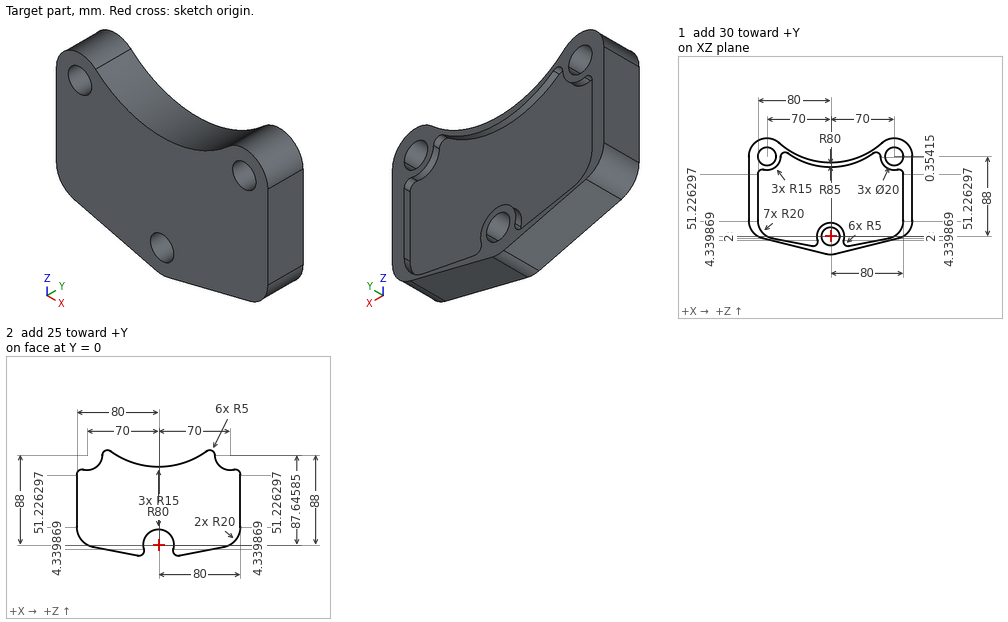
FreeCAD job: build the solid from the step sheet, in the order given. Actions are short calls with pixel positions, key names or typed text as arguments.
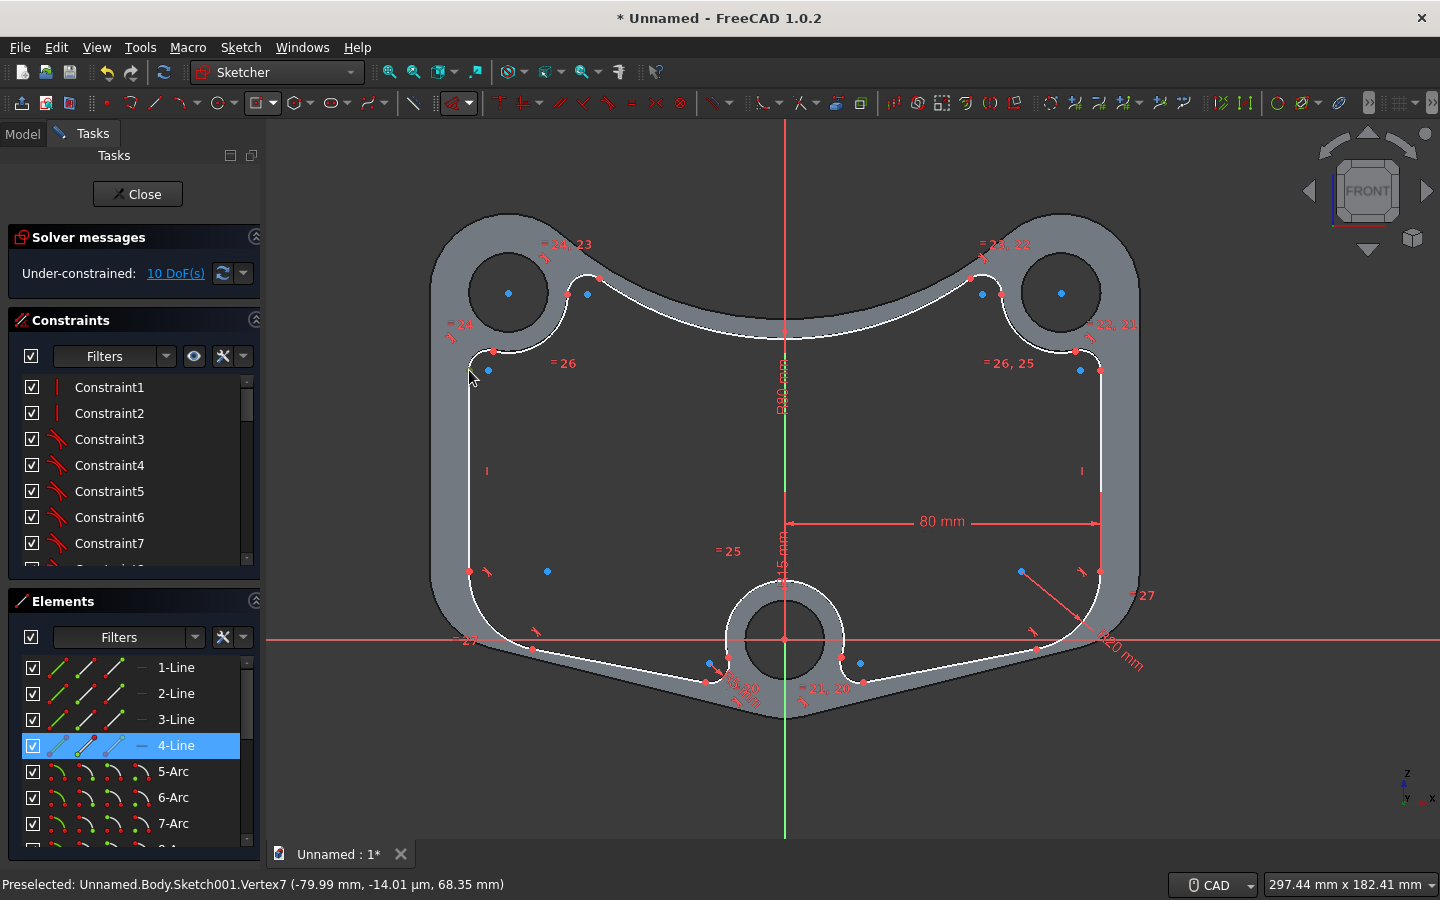
click(472, 104)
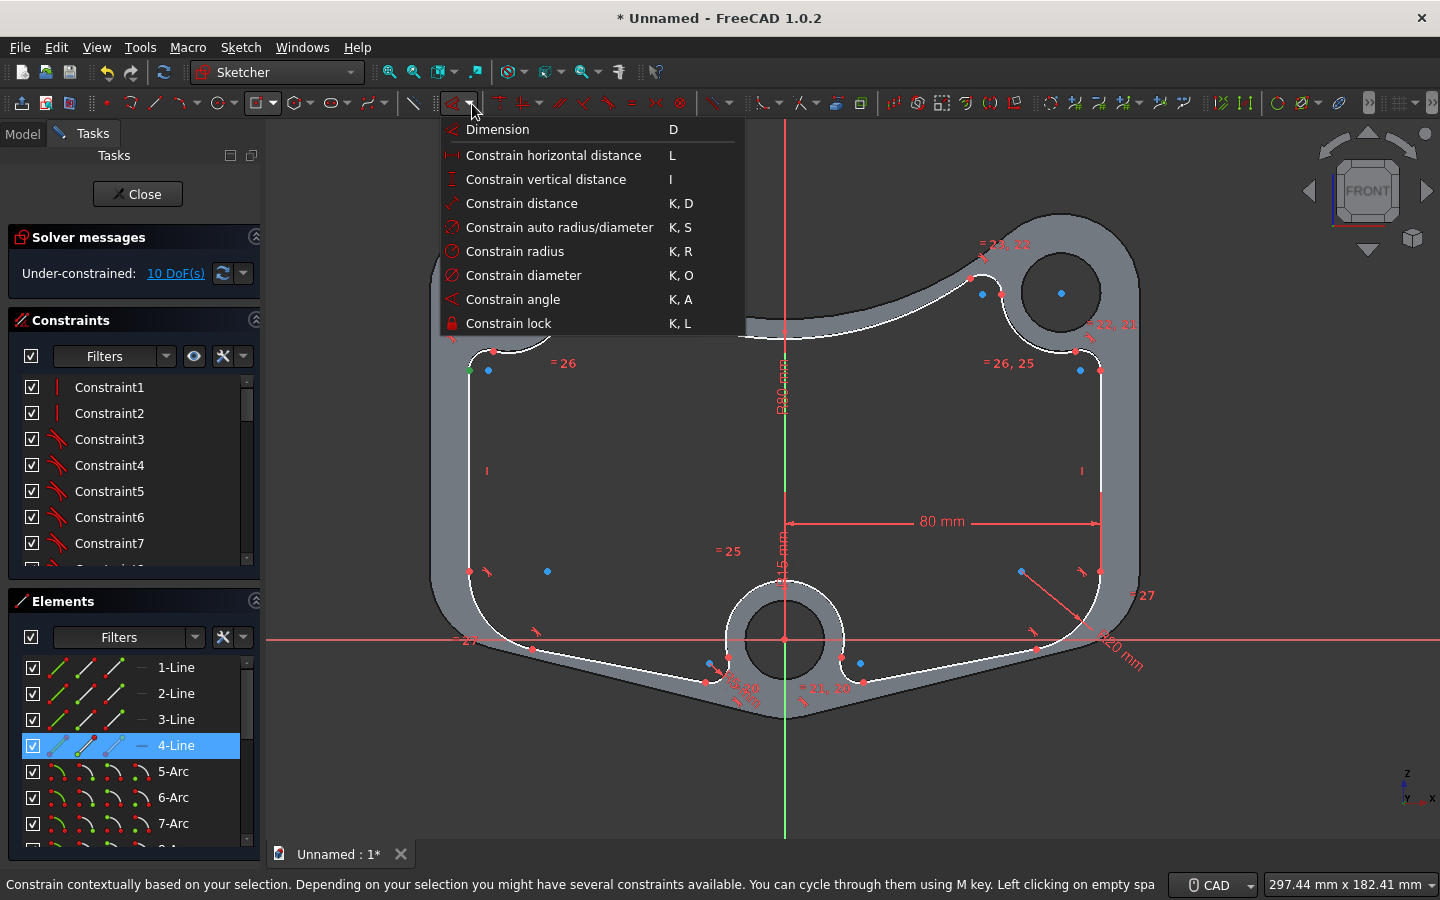
click(593, 155)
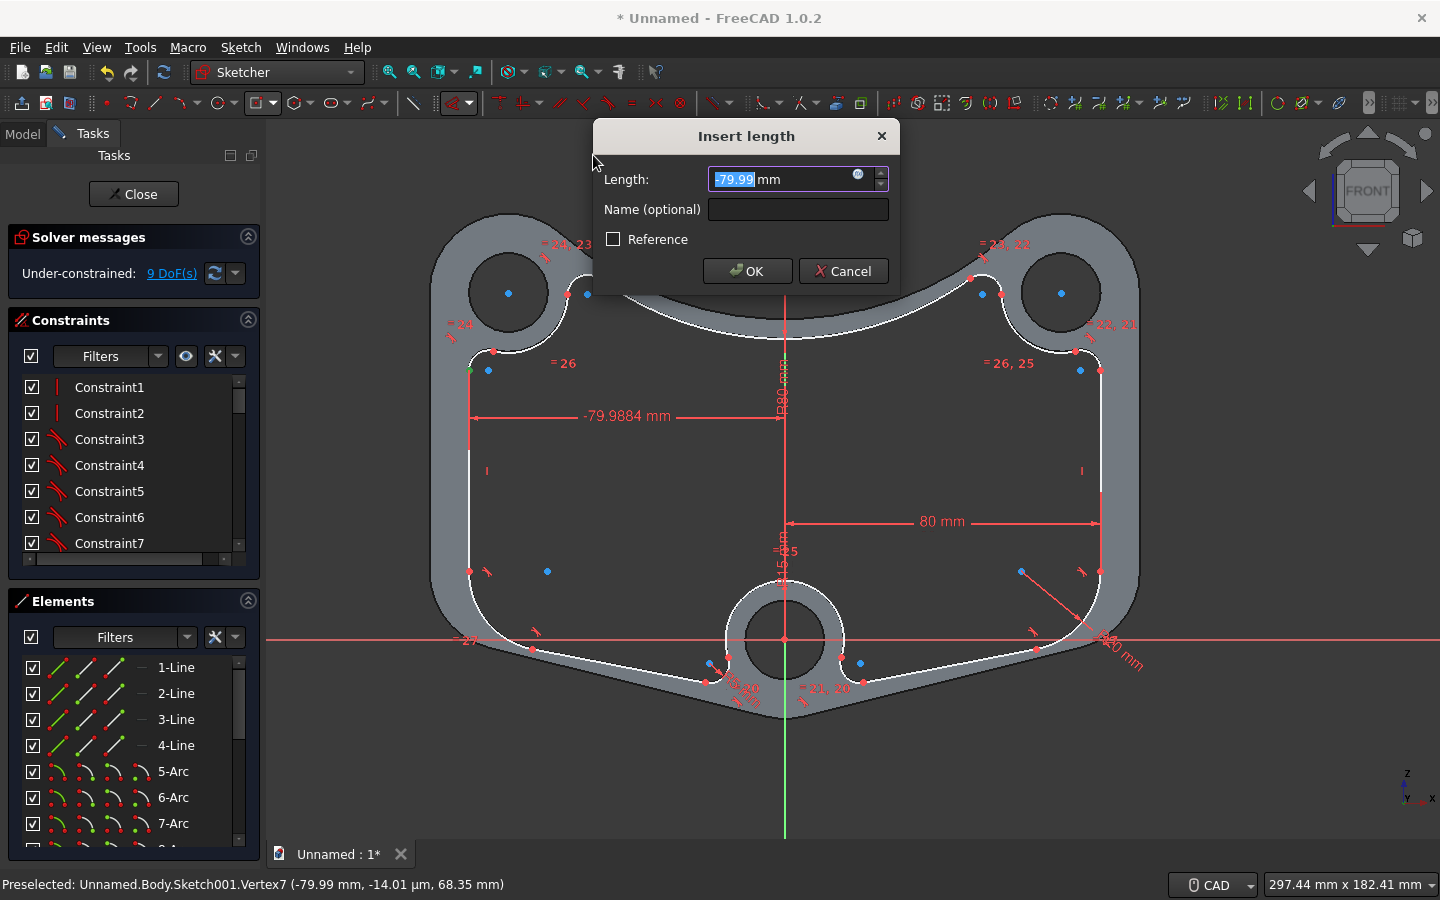
text(-80)
key(Return)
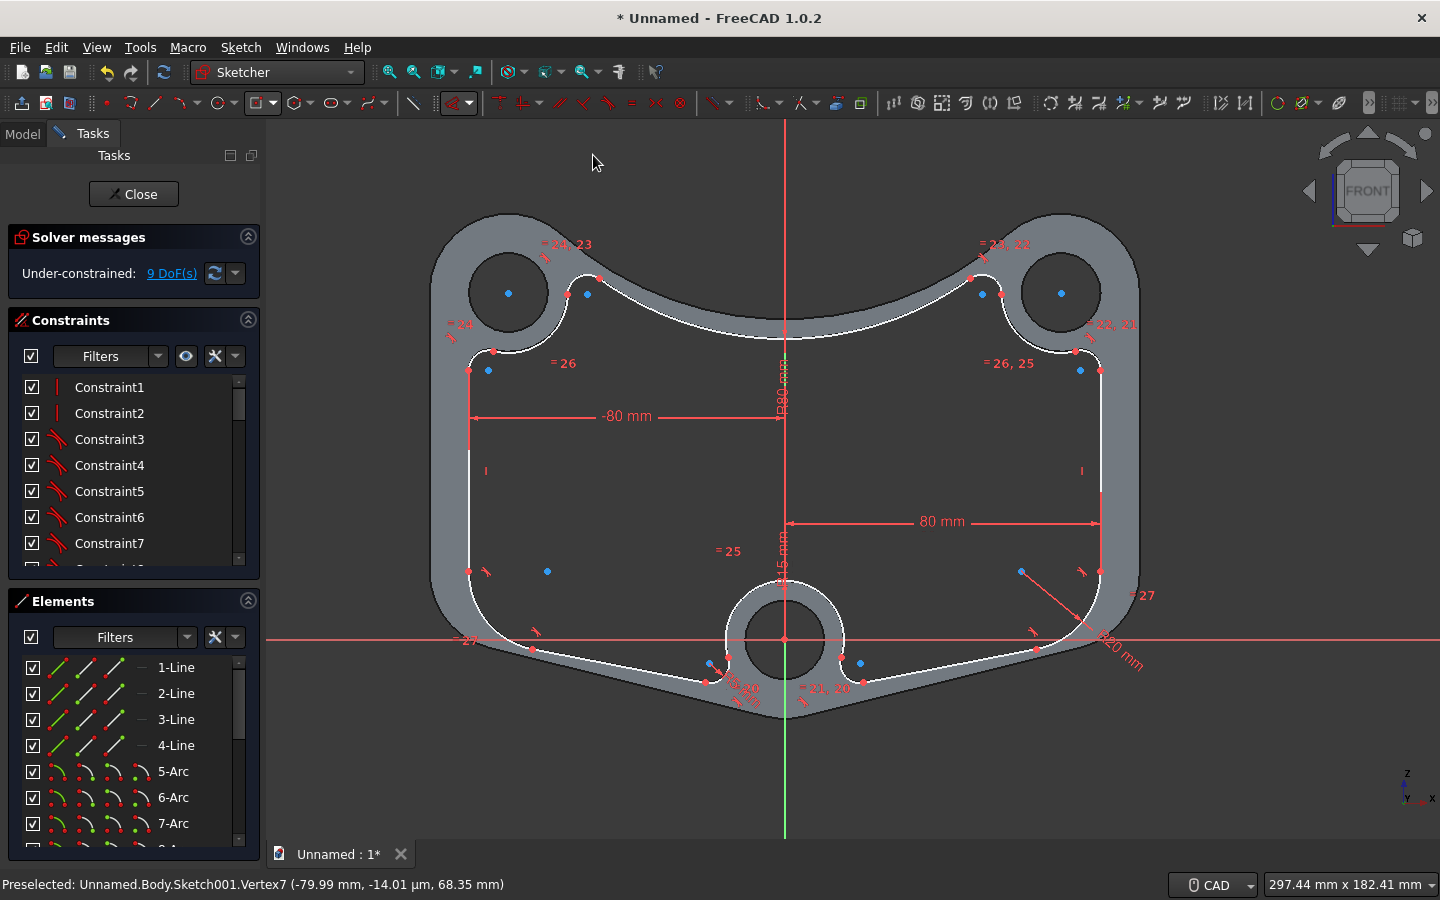
click(1061, 294)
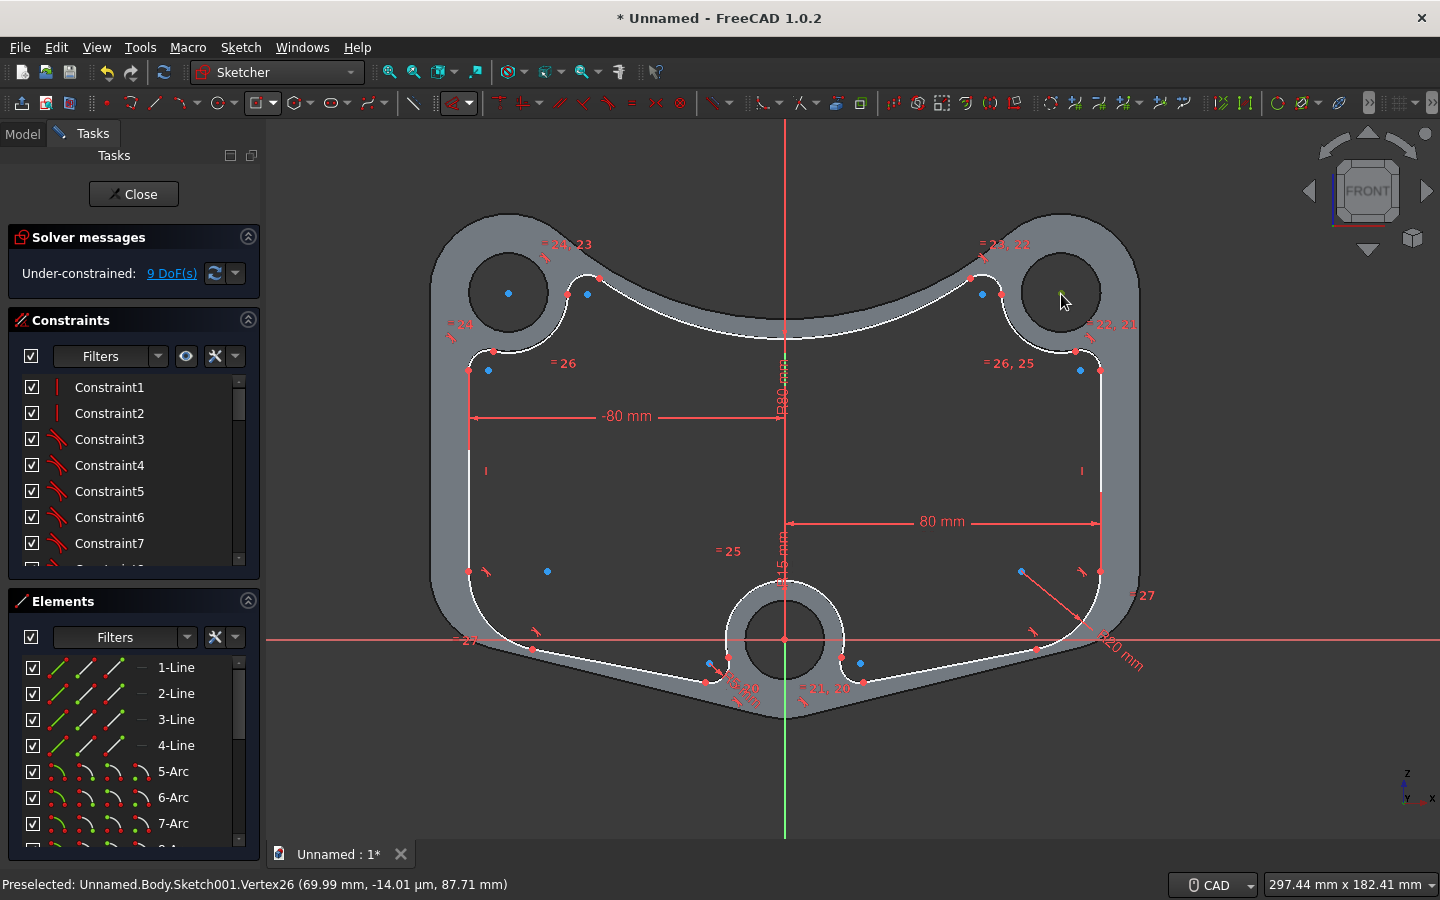
key(l)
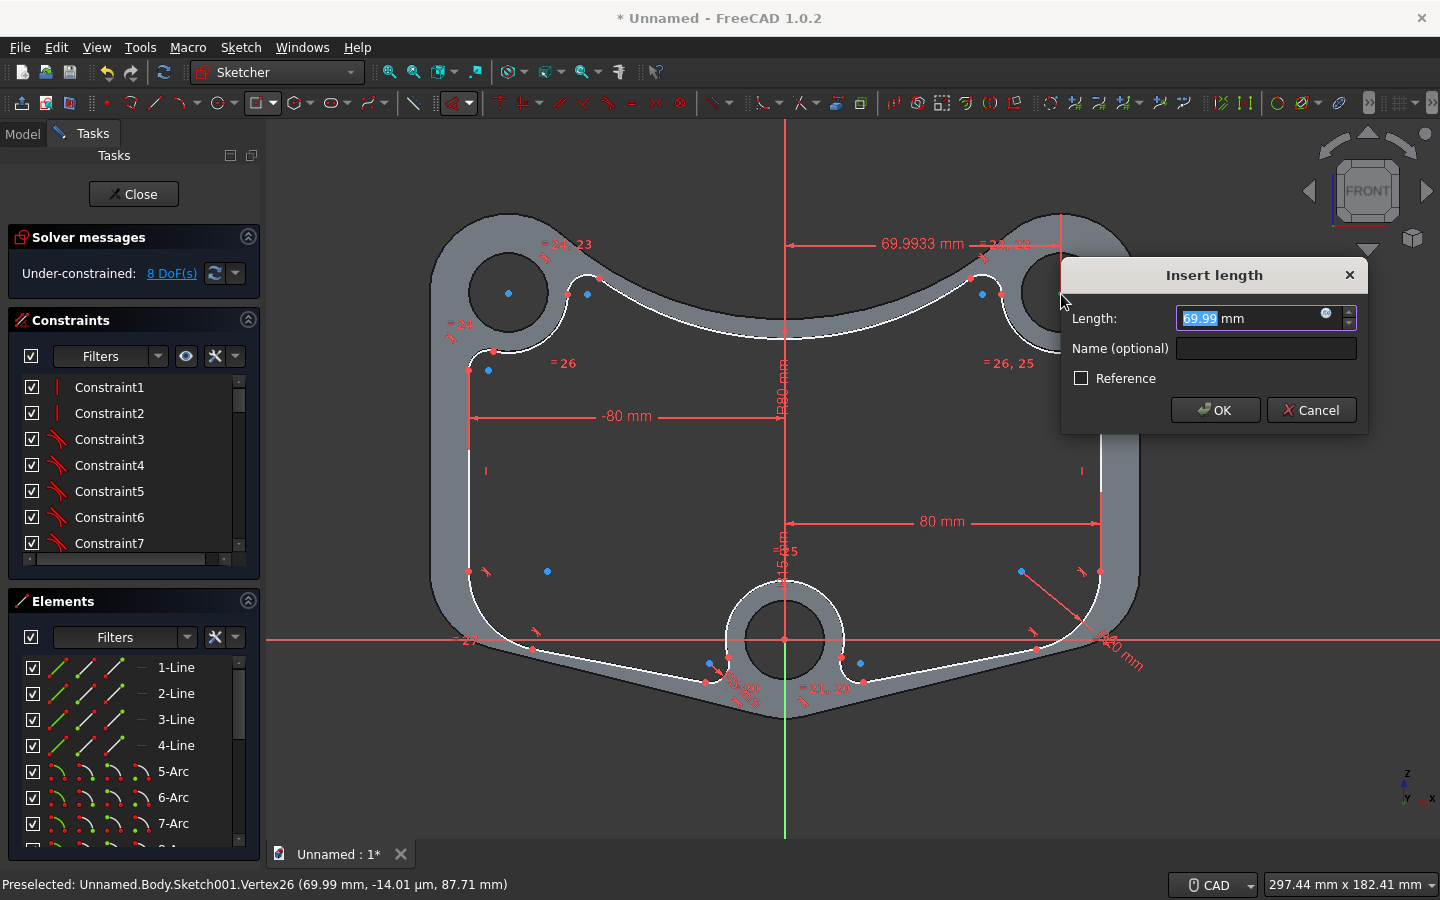
text(70)
key(Return)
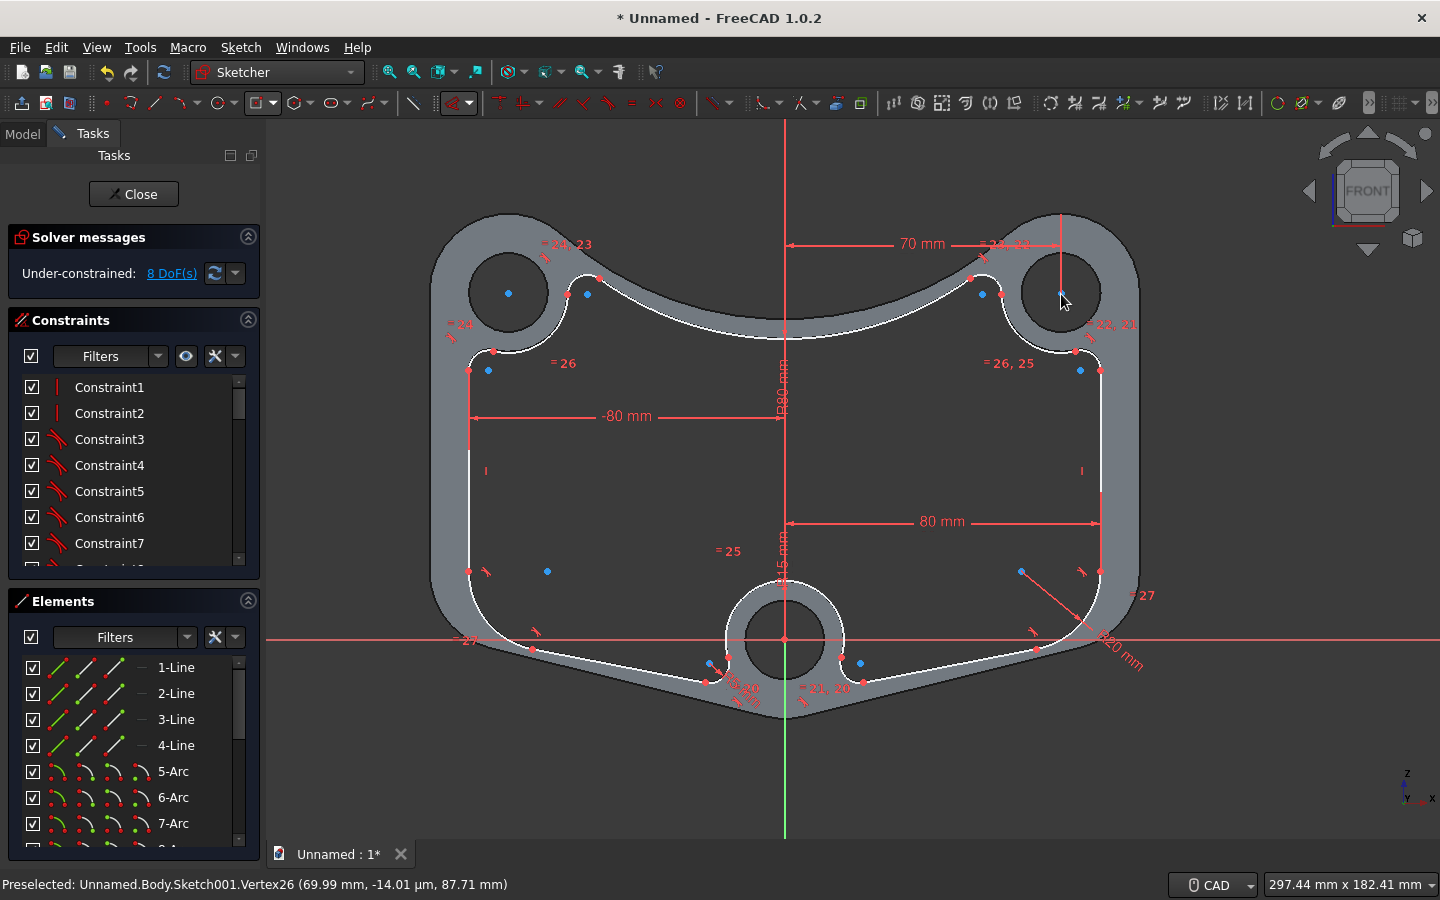
click(1061, 294)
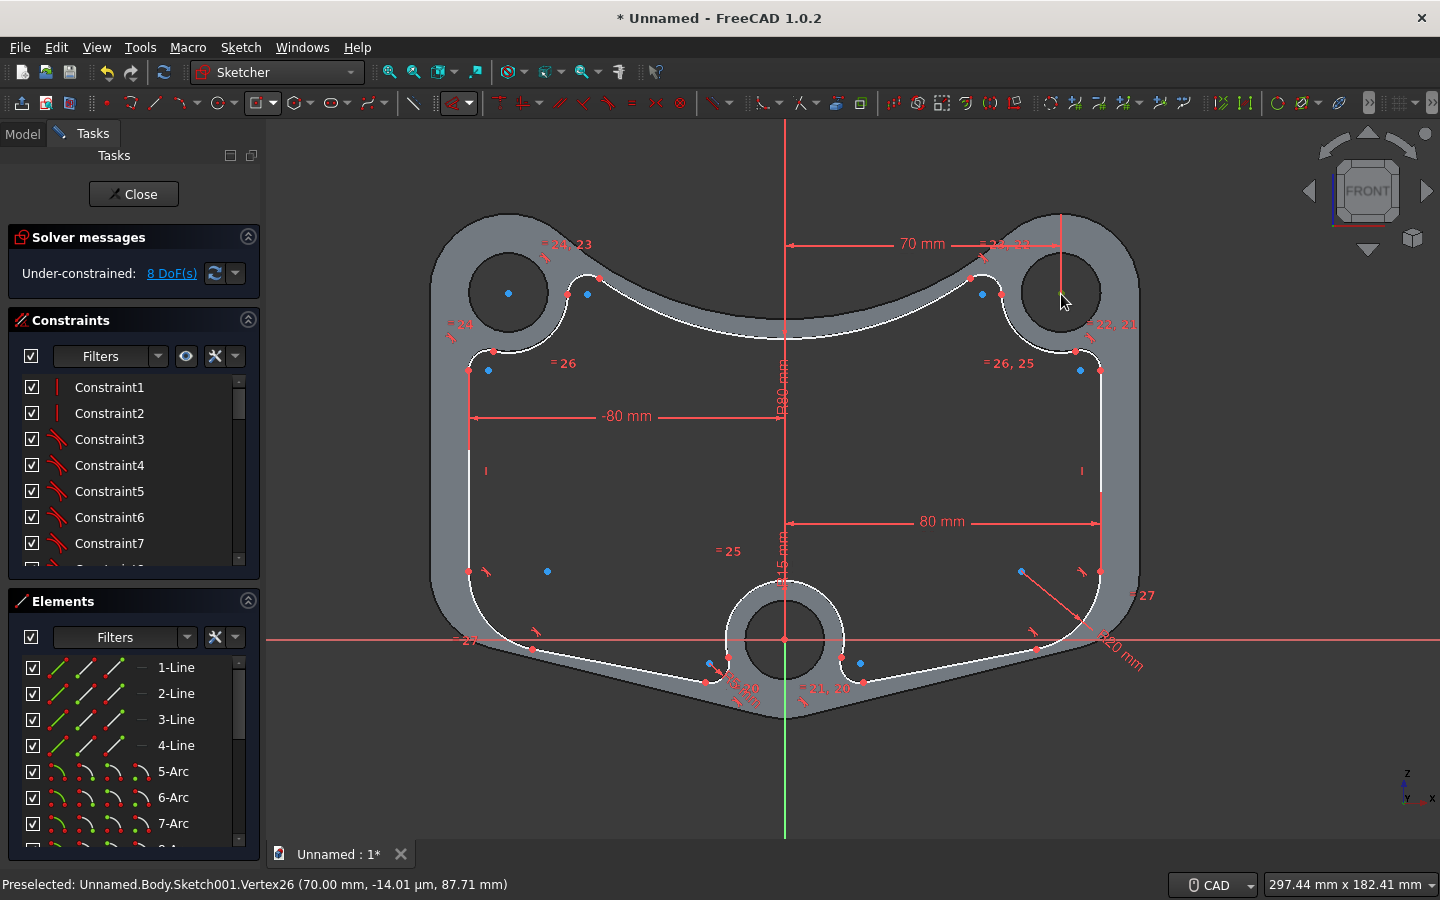
key(i)